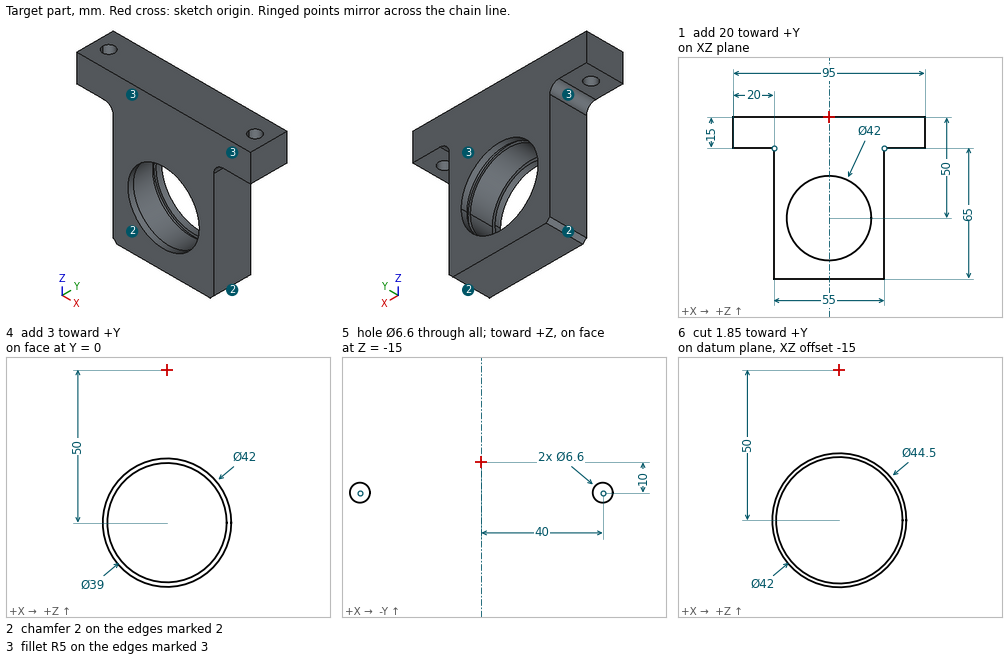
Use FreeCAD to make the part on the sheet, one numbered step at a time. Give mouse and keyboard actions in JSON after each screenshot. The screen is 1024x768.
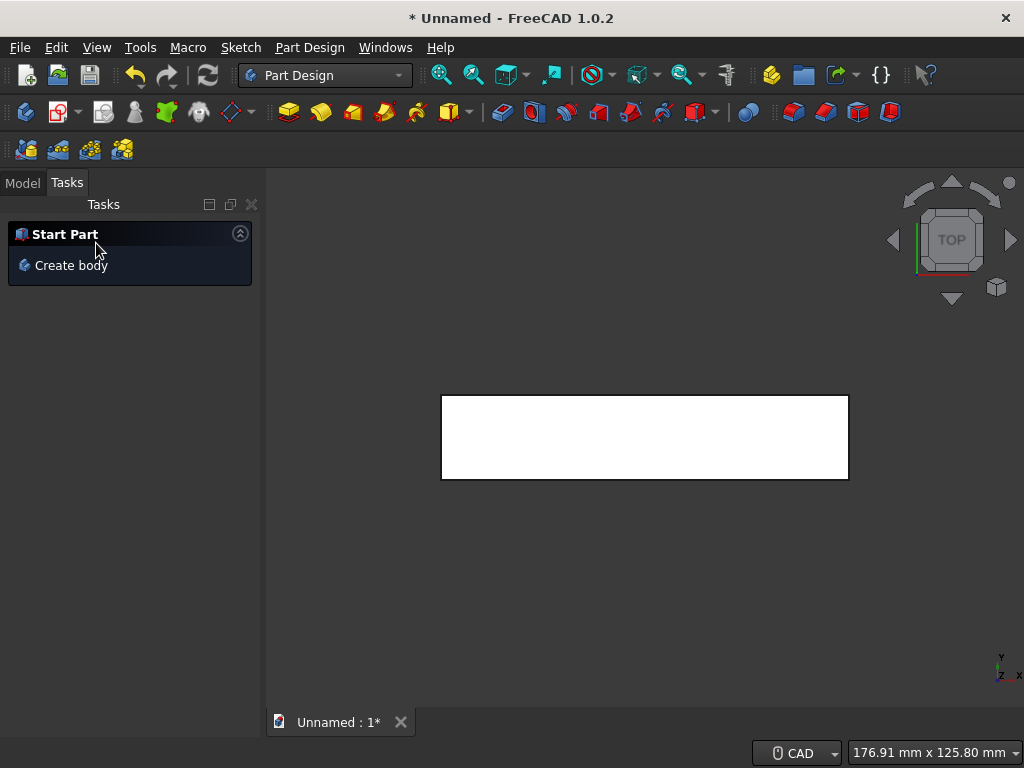
{"action": "key", "text": "1"}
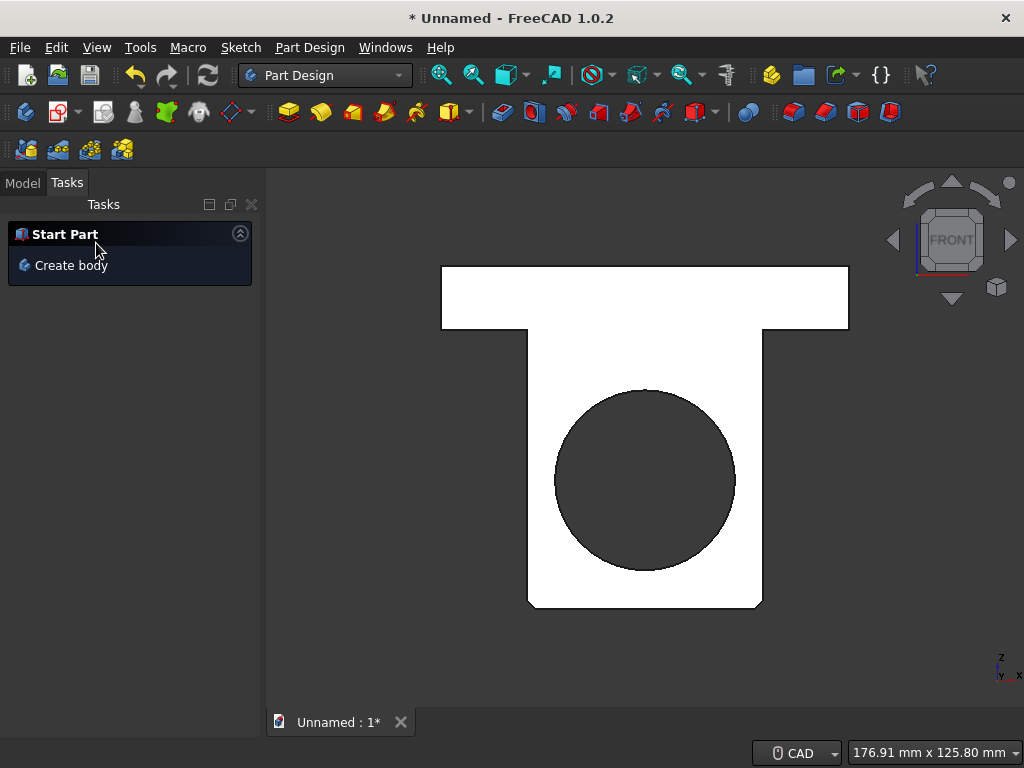
{"action": "key", "text": "3"}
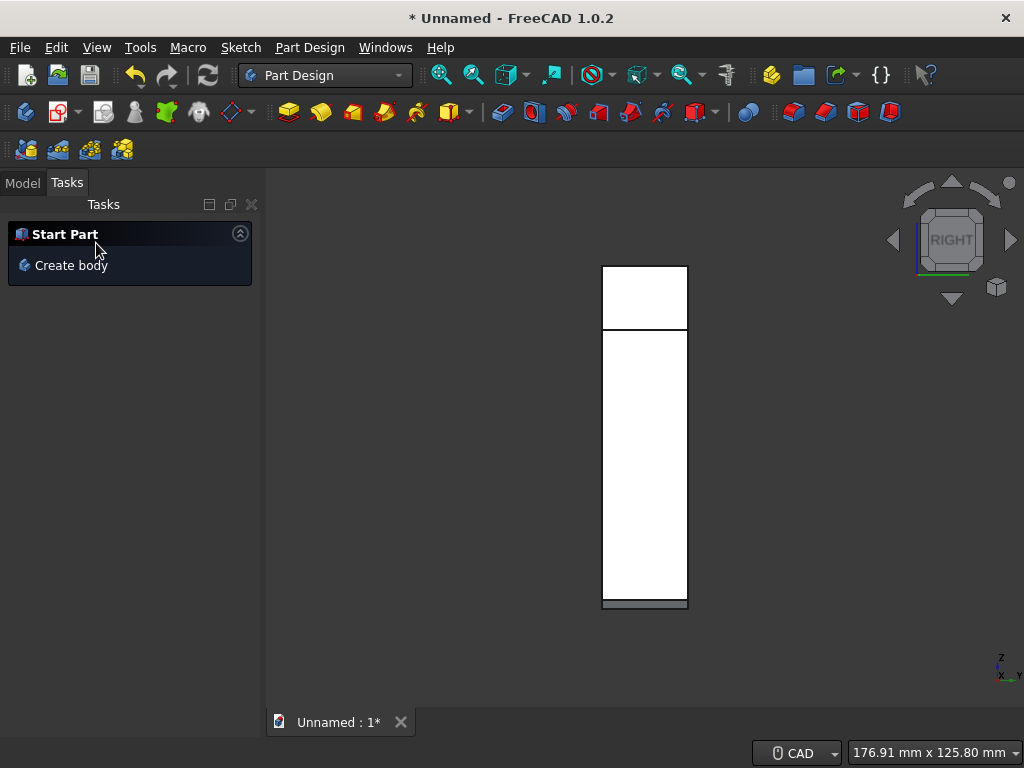
{"action": "key", "text": "5"}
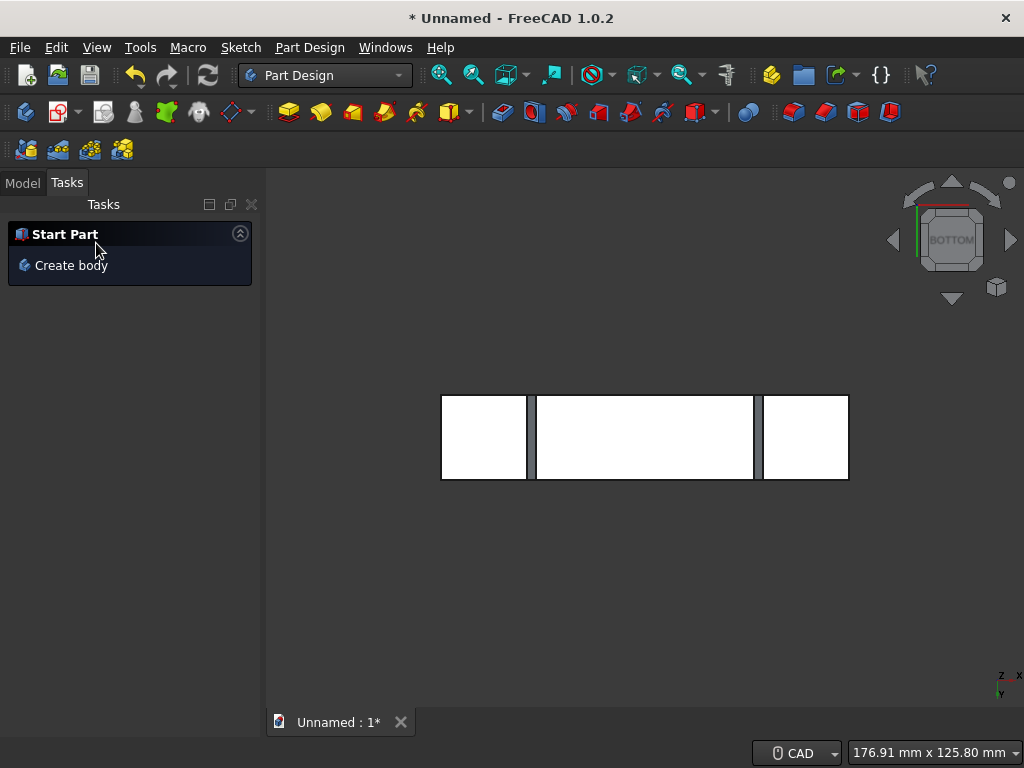
{"action": "key", "text": "4"}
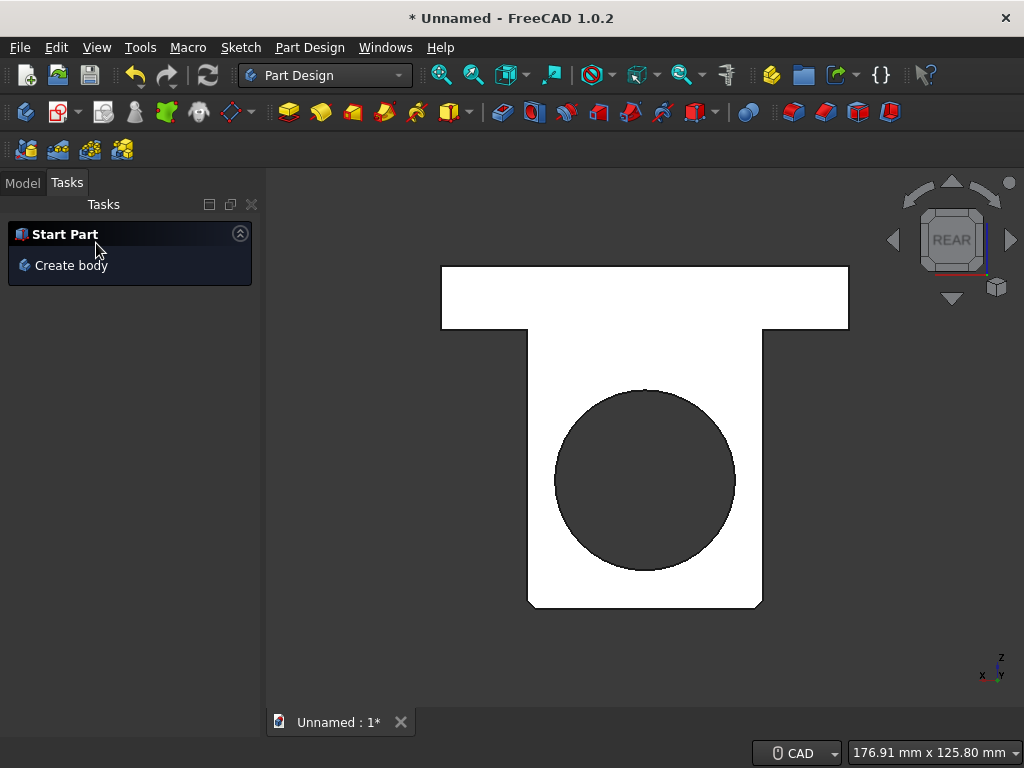
{"action": "key", "text": "6"}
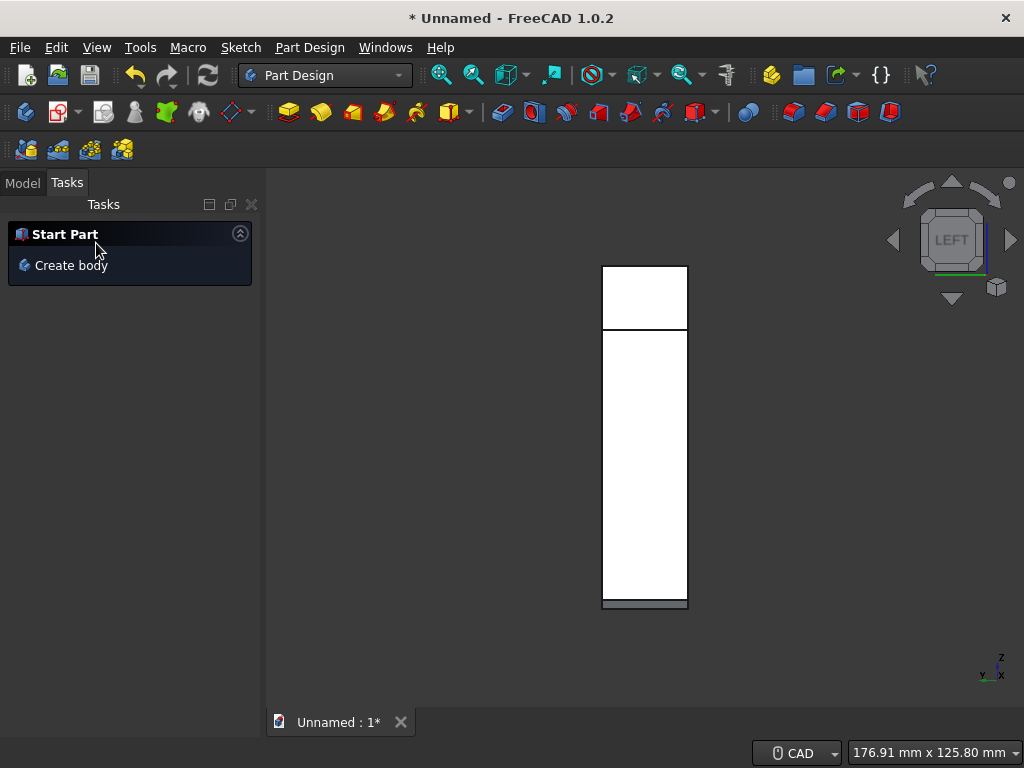
{"action": "key", "text": "v 3"}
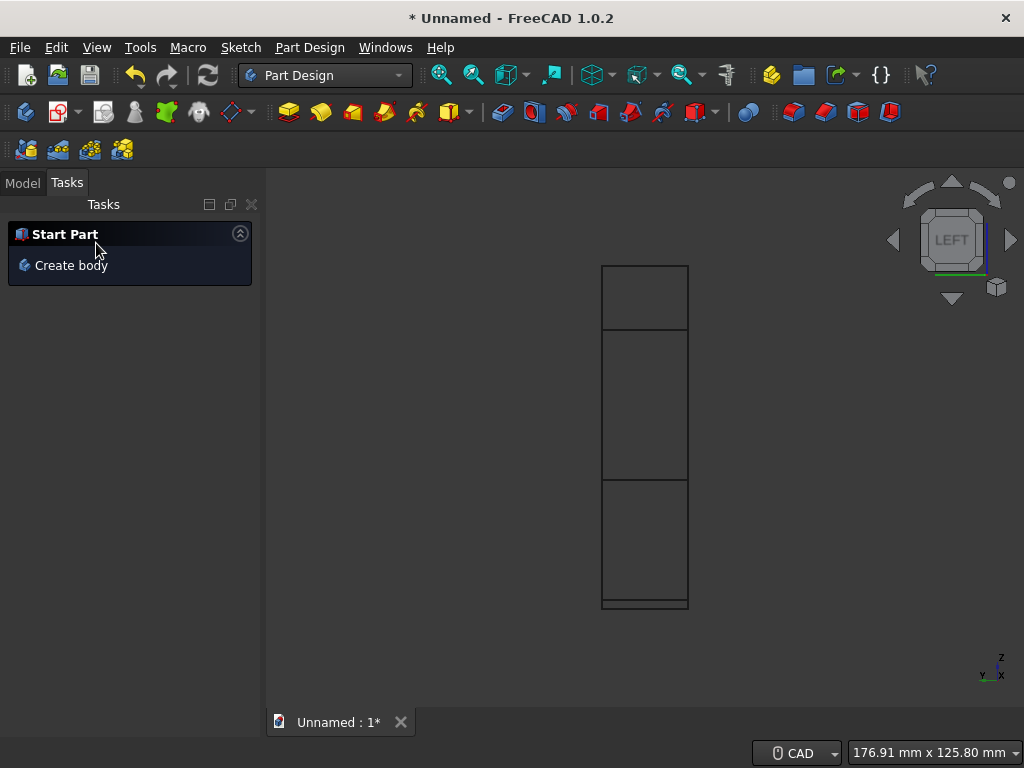
{"action": "key", "text": "0"}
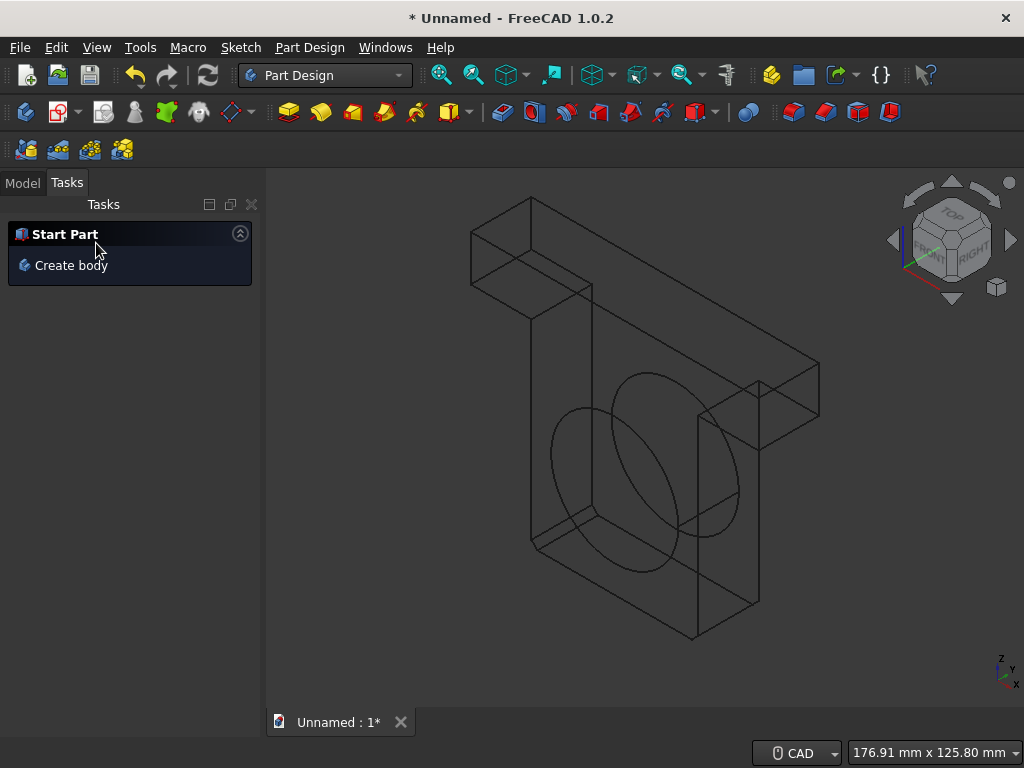
{"action": "left_click", "coordinate": [562, 301]}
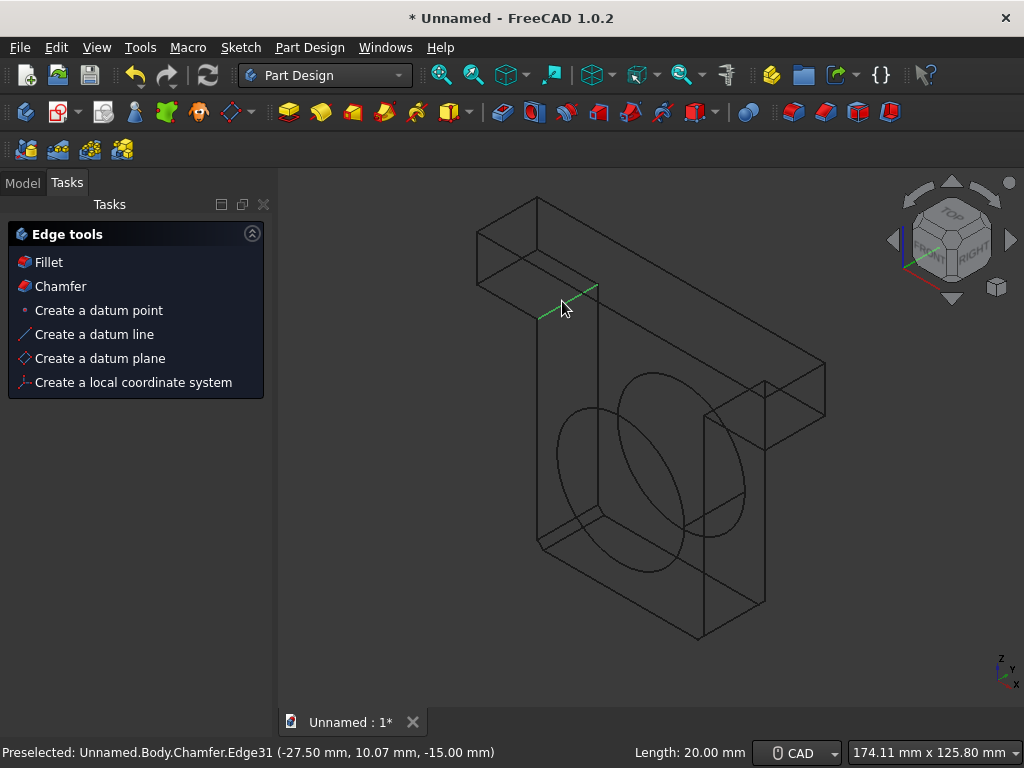
{"action": "left_click", "coordinate": [734, 397], "text": "ctrl"}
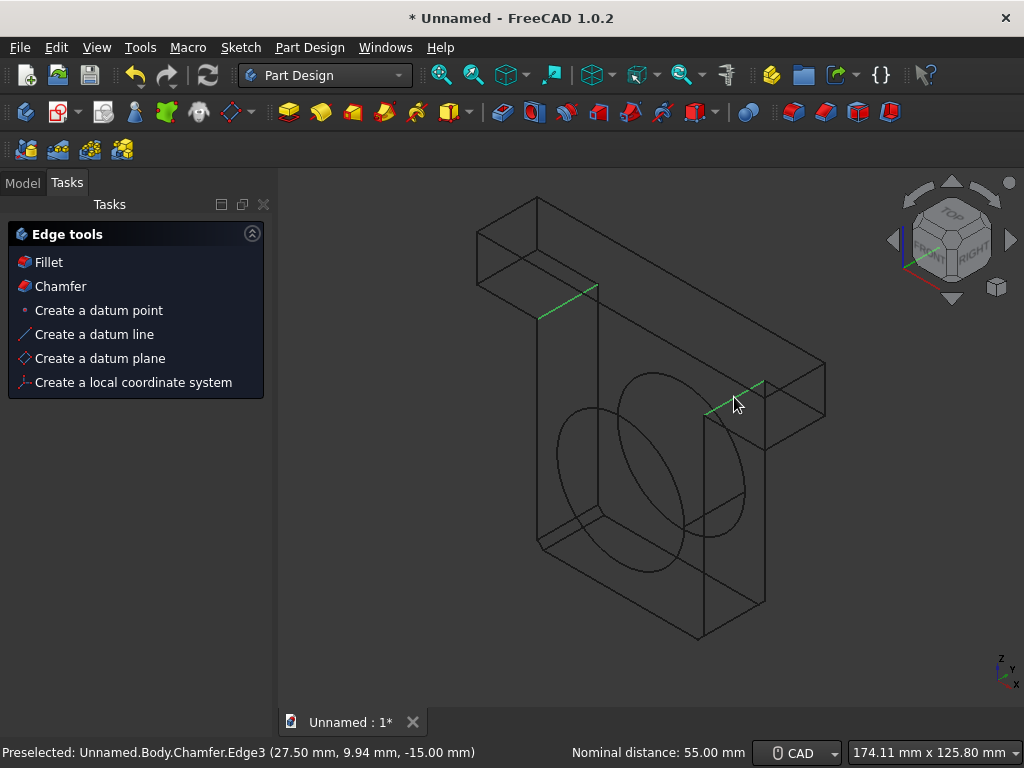
{"action": "key", "text": "v 1"}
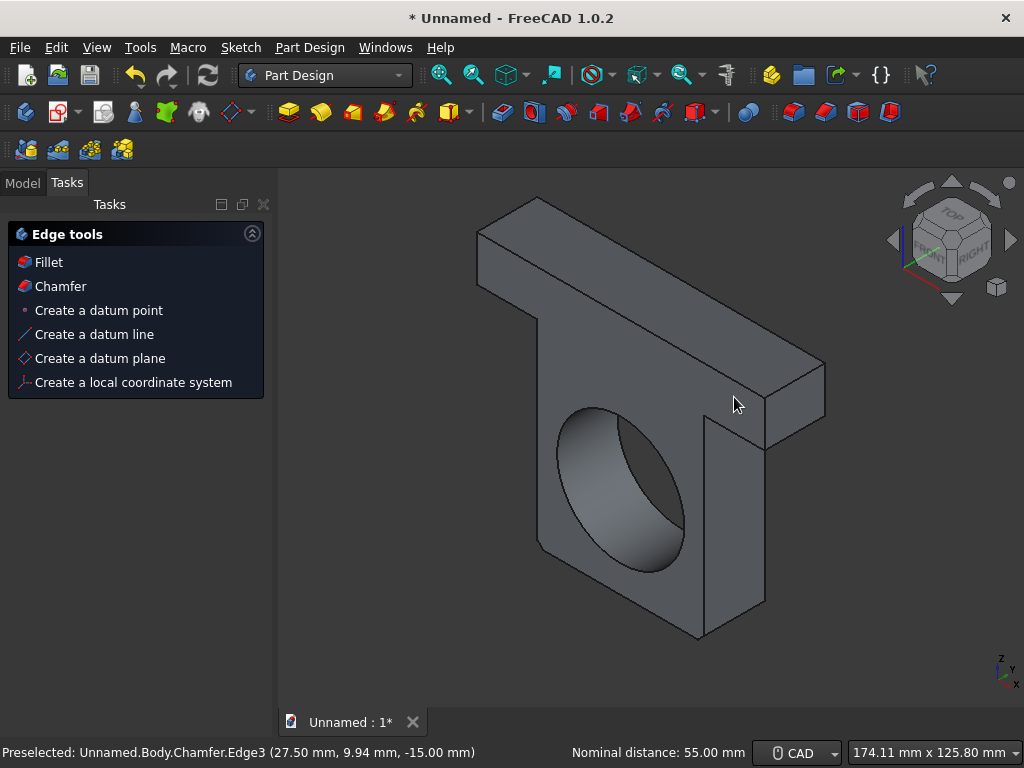
{"action": "left_click", "coordinate": [794, 112]}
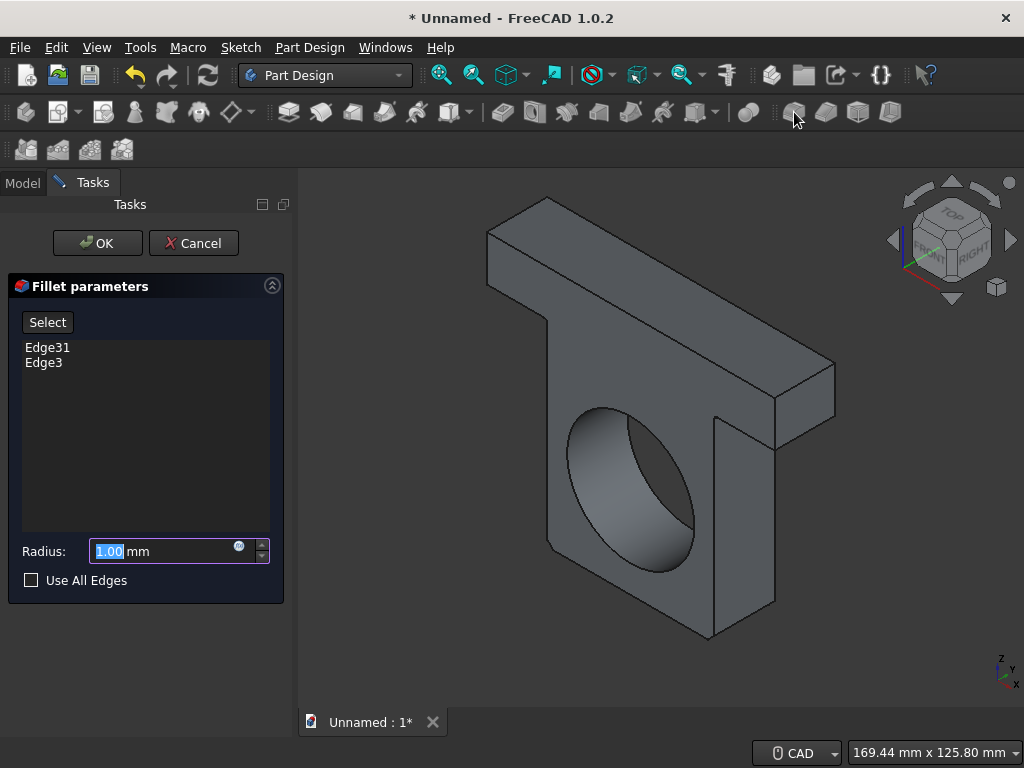
{"action": "type", "text": "5"}
{"action": "key", "text": "Tab"}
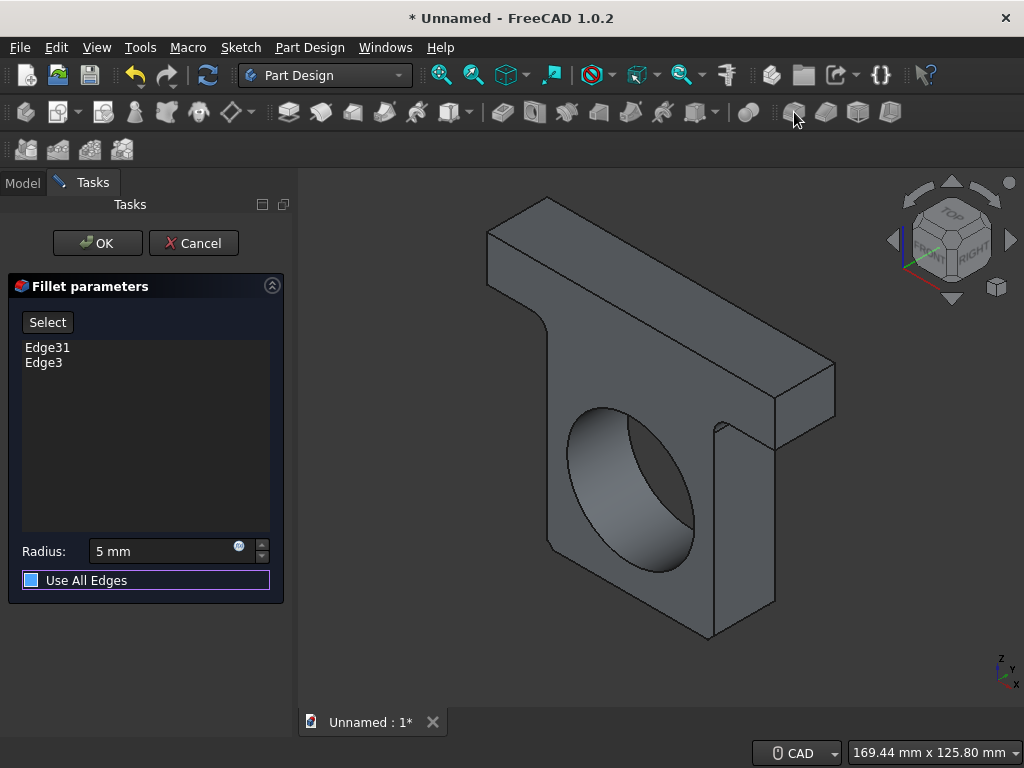
{"action": "left_click", "coordinate": [98, 243]}